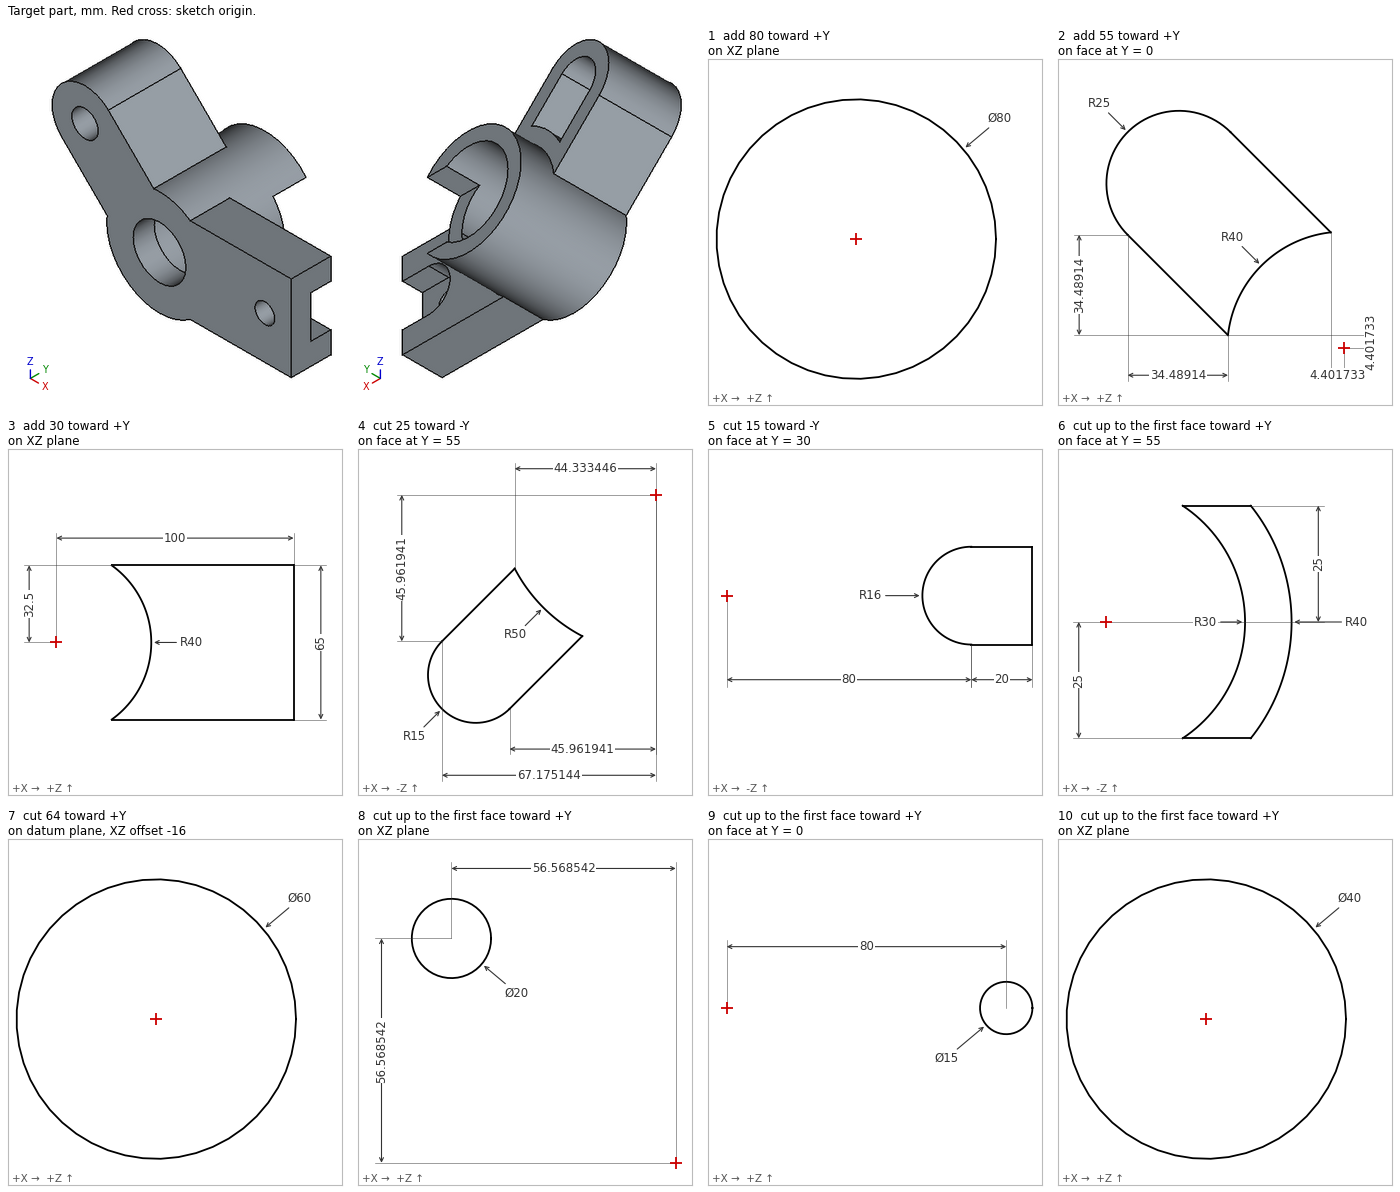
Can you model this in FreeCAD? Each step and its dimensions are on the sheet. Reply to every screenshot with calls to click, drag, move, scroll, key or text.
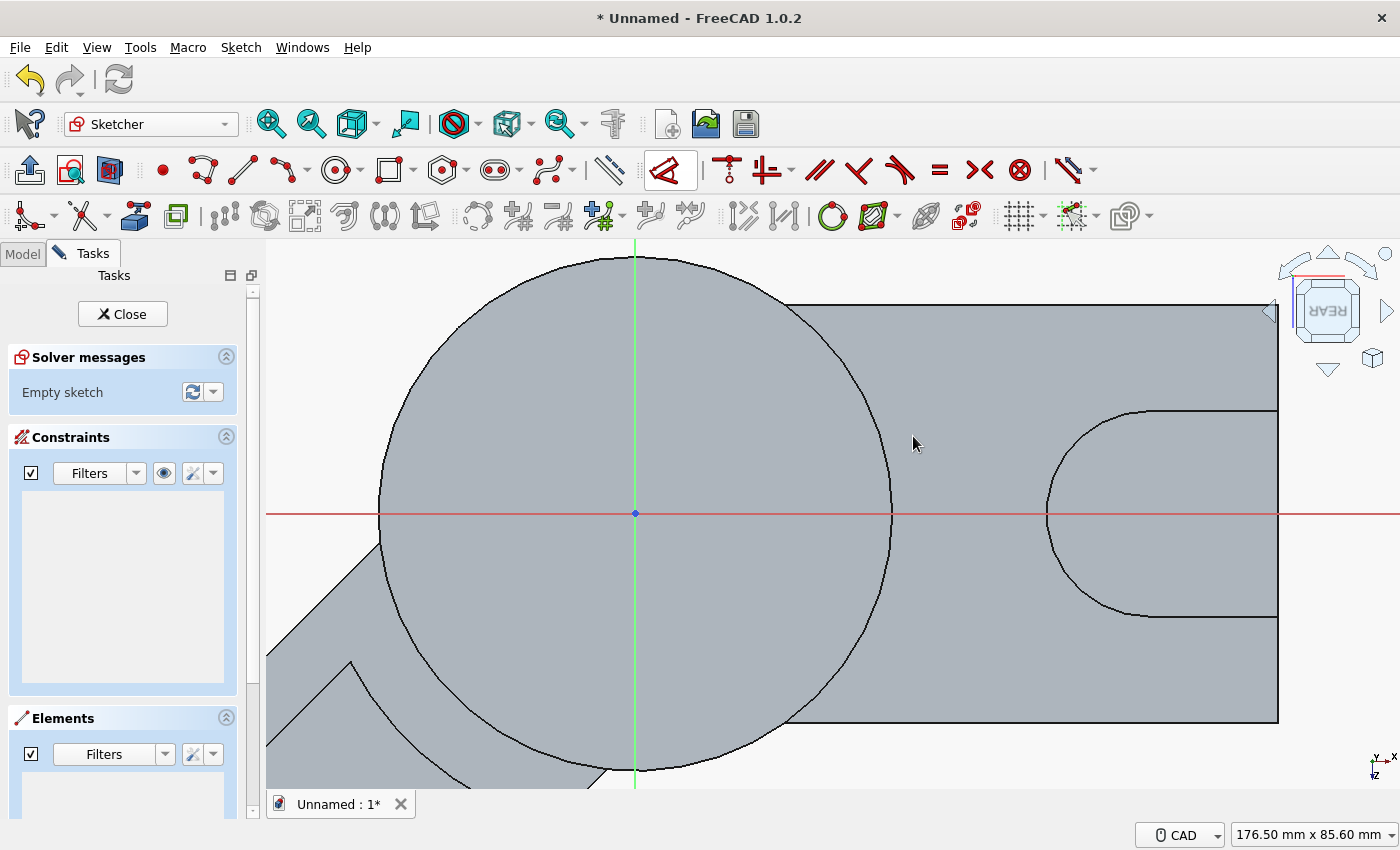
click(244, 170)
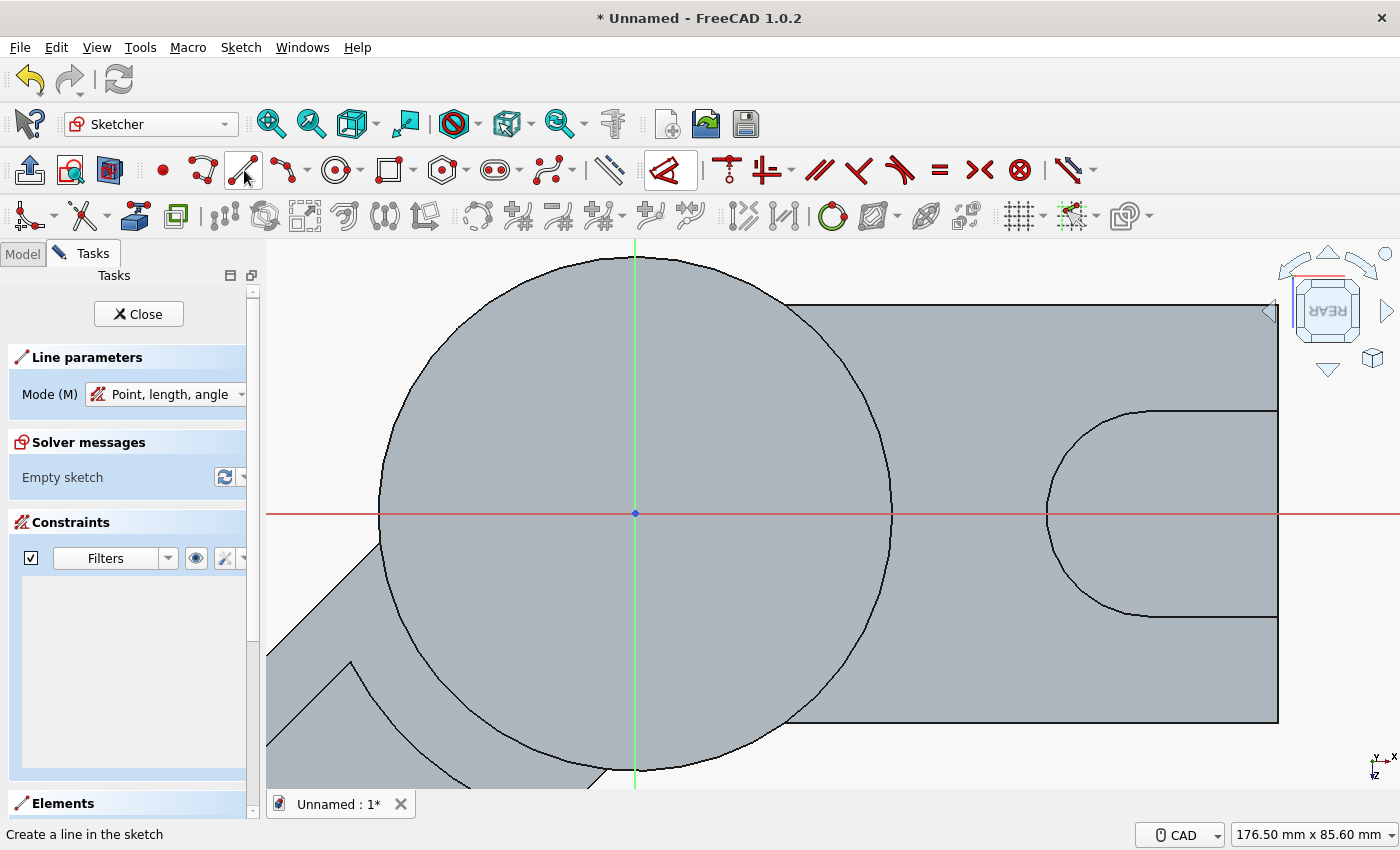
click(836, 353)
click(742, 353)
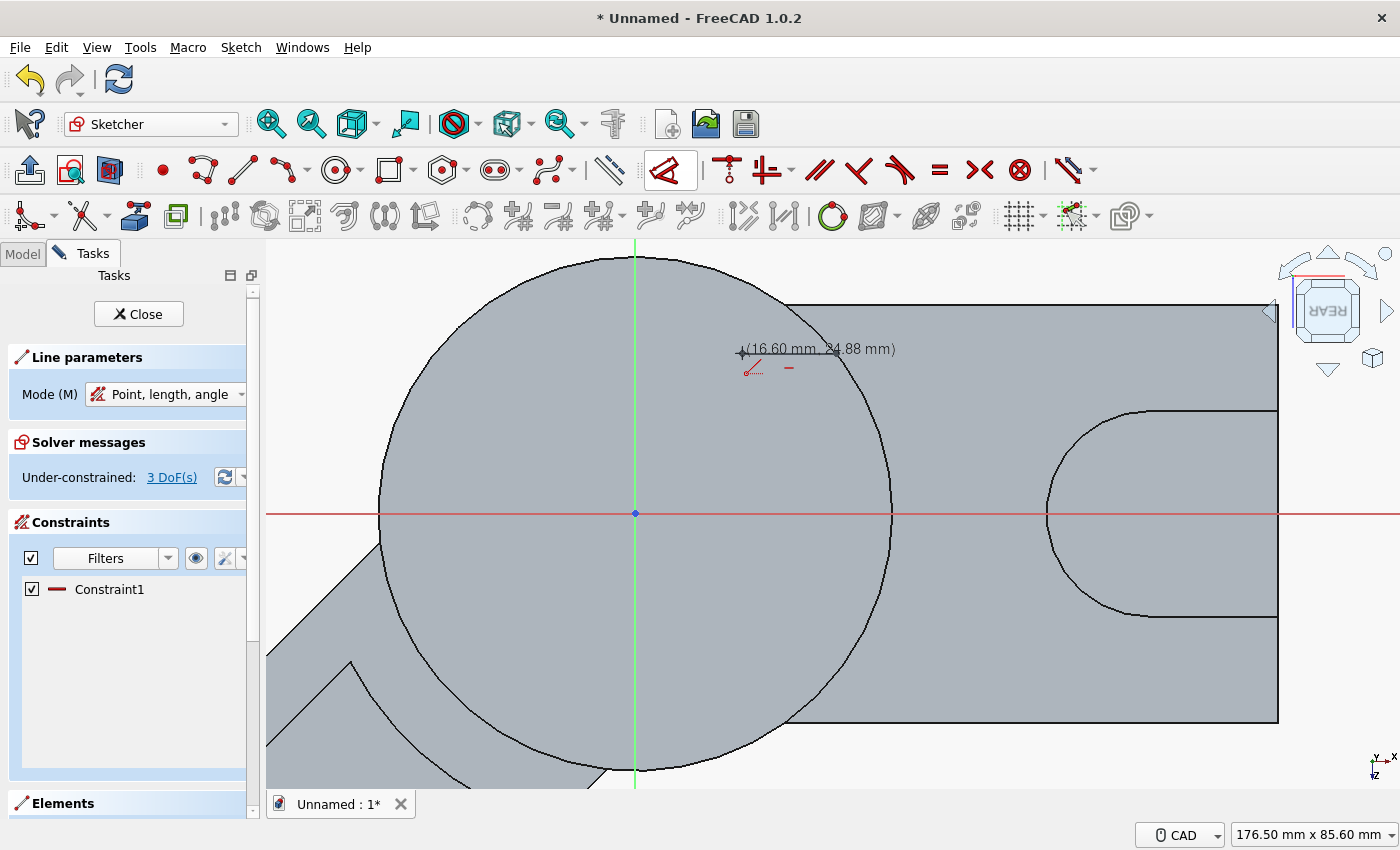
click(742, 674)
click(836, 674)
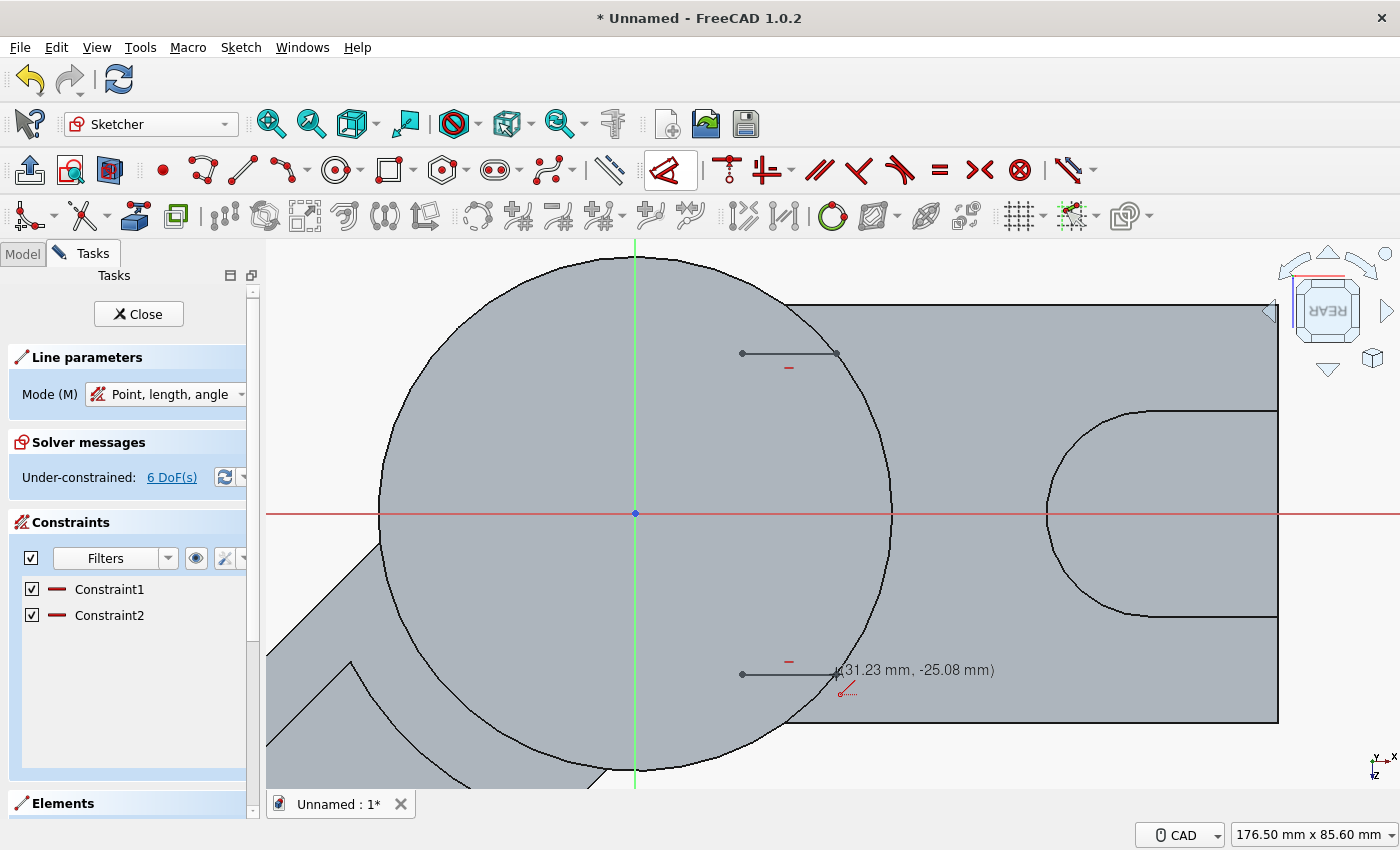
click(284, 170)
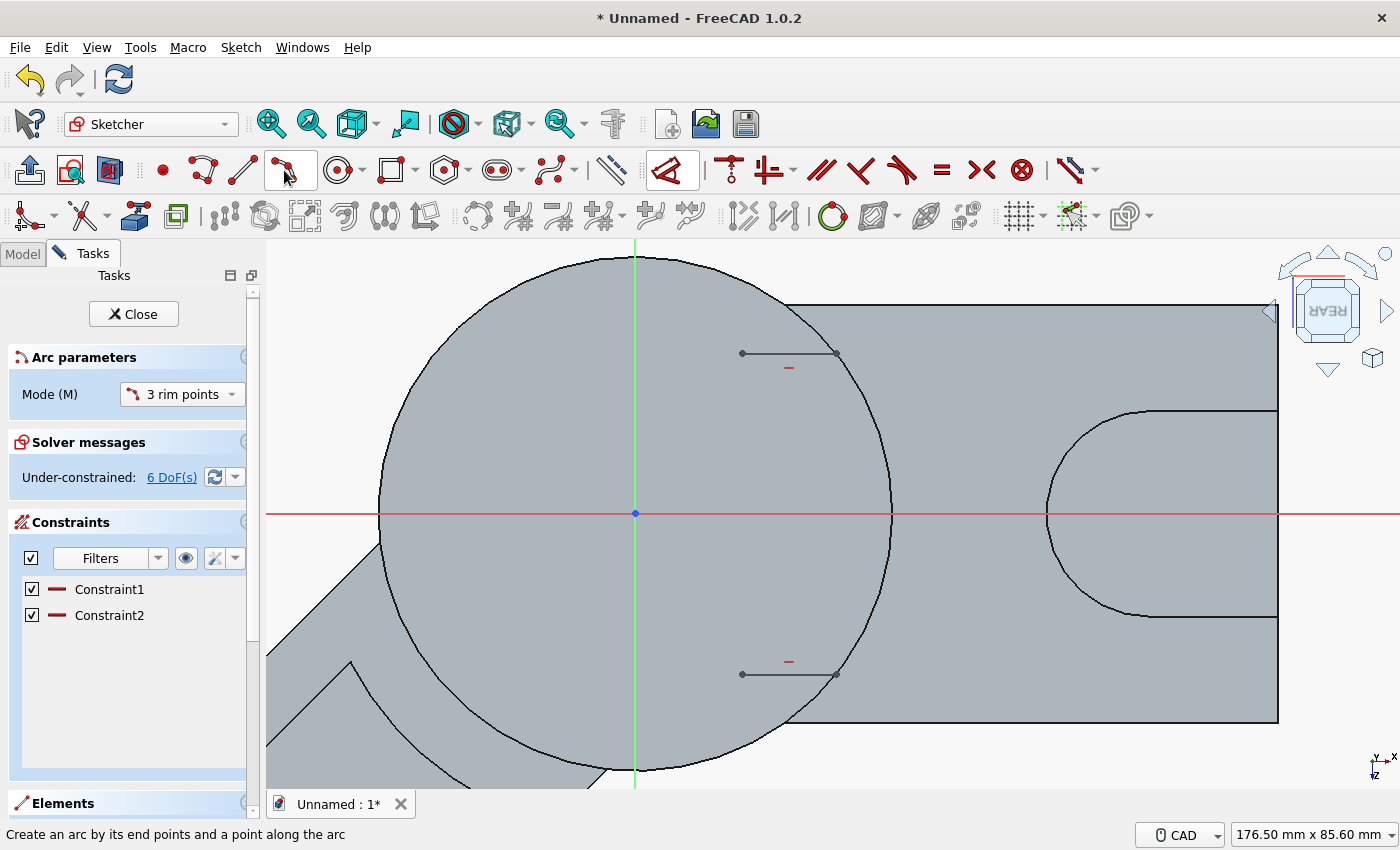
click(742, 354)
click(742, 675)
click(824, 552)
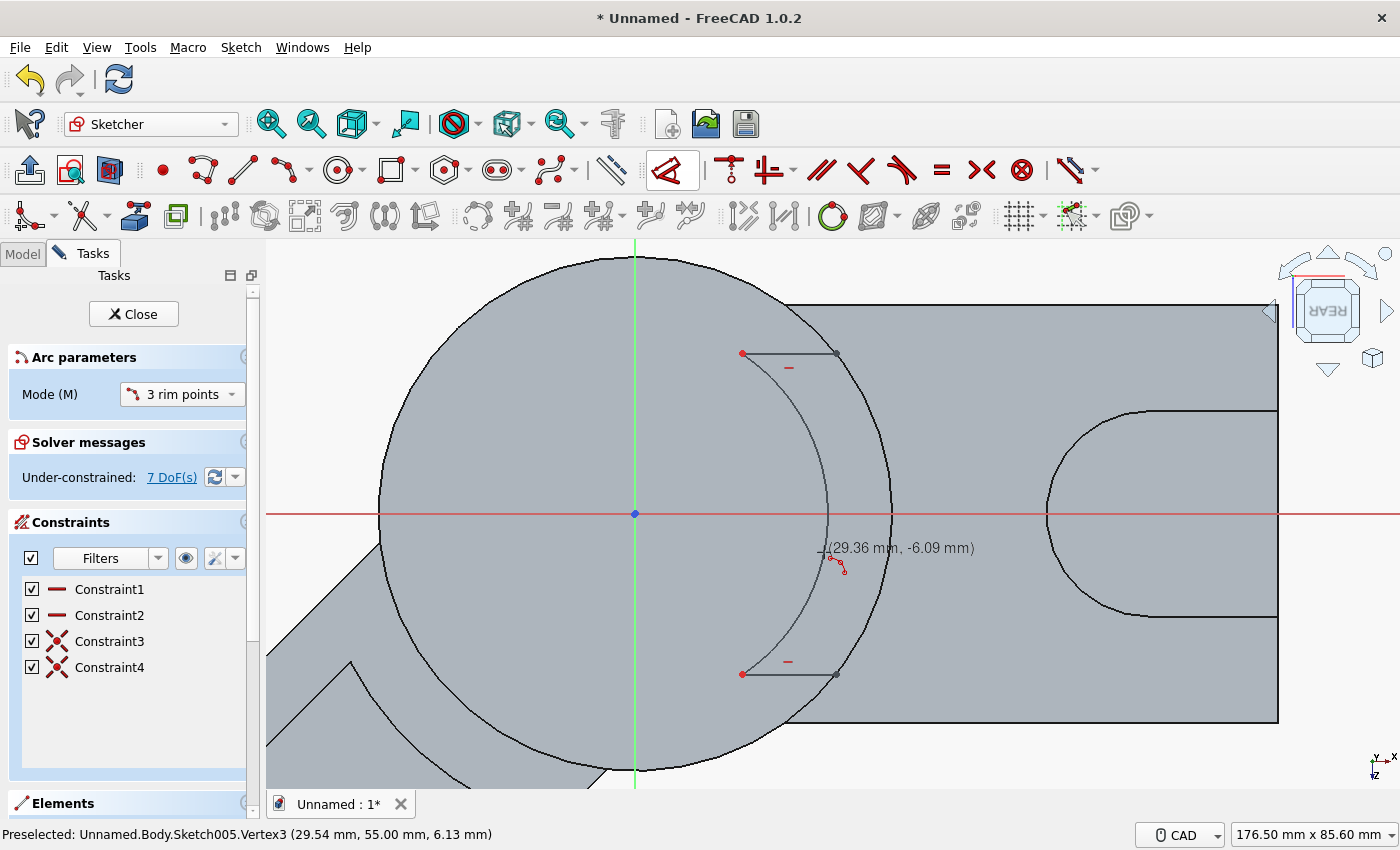
click(836, 675)
click(836, 354)
click(890, 548)
key(Escape)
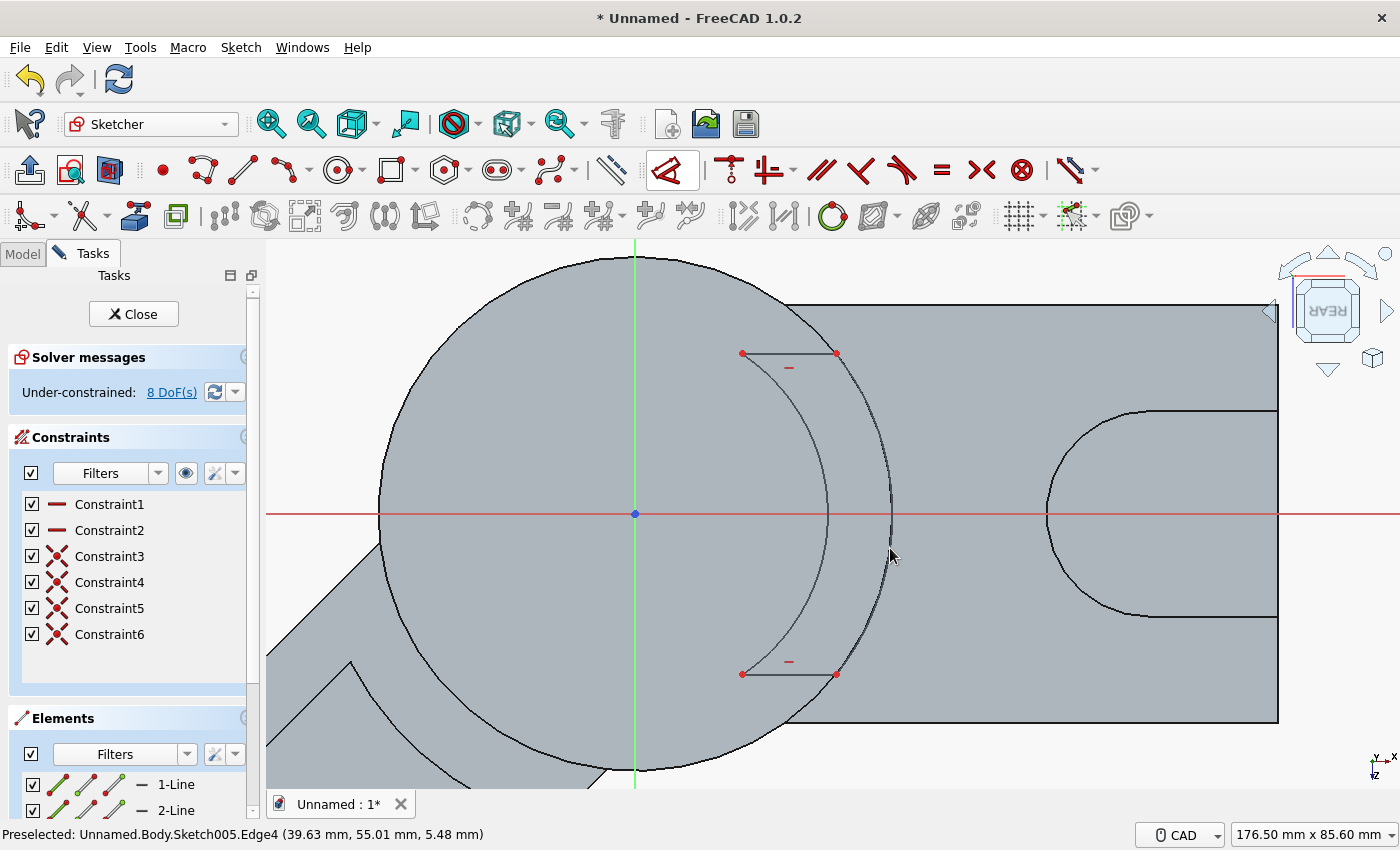
click(813, 588)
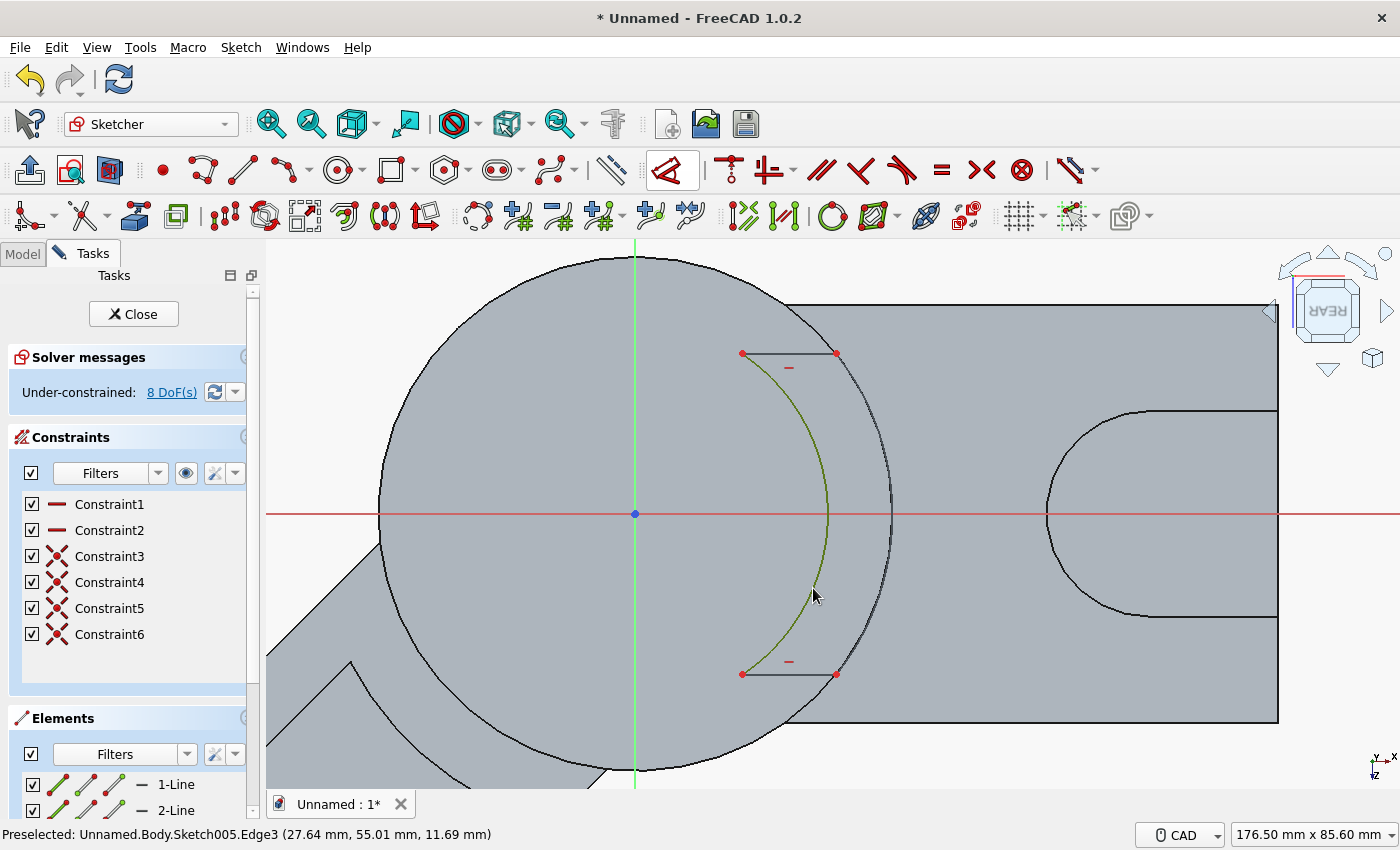
click(883, 583)